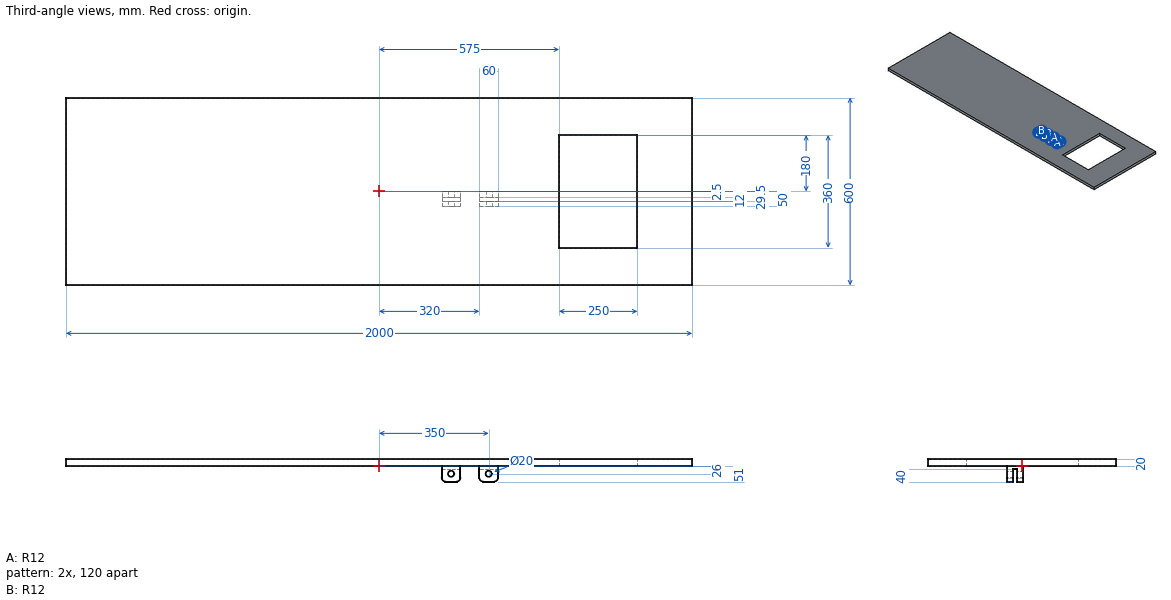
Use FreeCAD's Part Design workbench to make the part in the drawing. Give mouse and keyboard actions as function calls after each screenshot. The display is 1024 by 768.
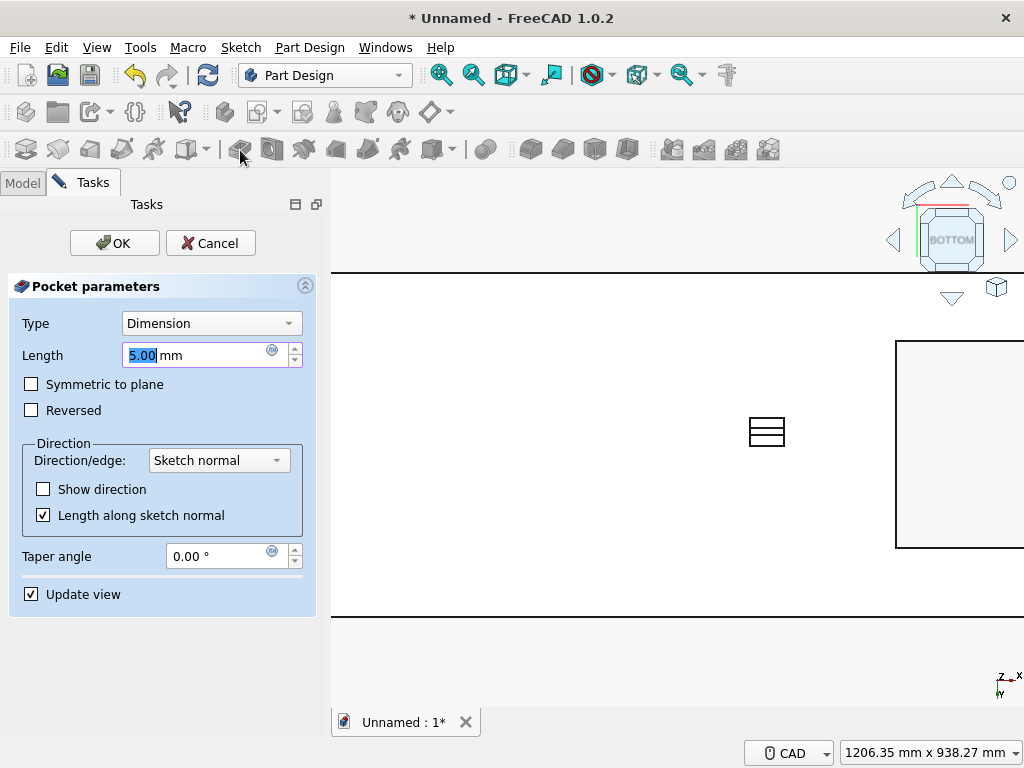
text(40)
key(Tab)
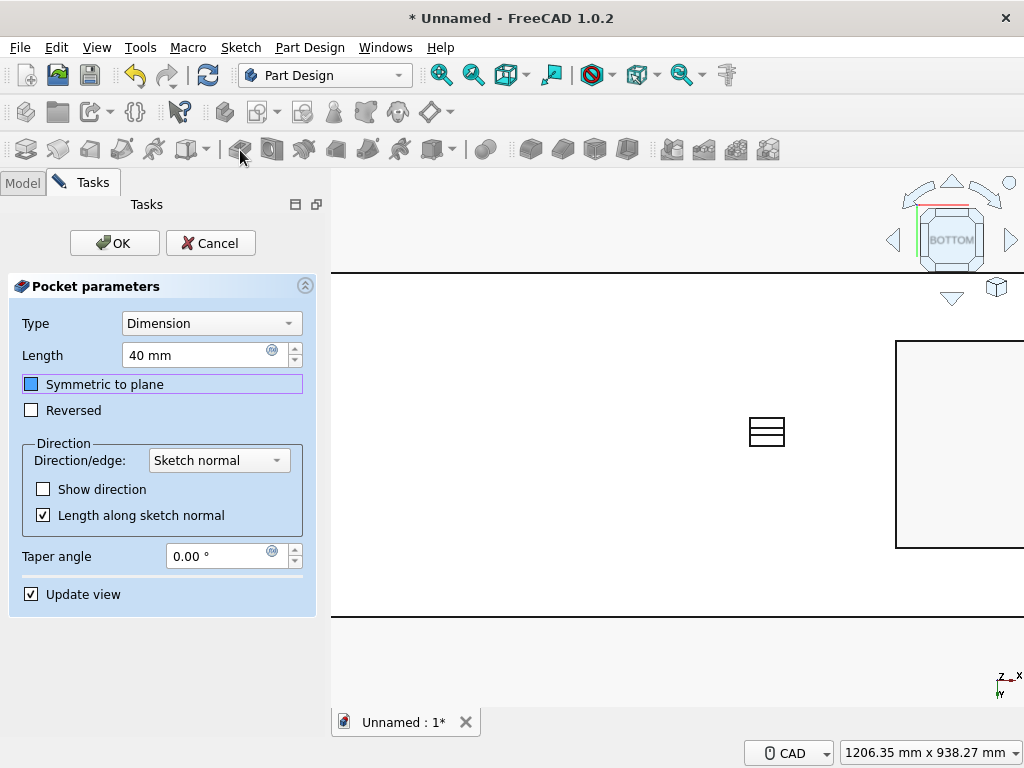
click(115, 243)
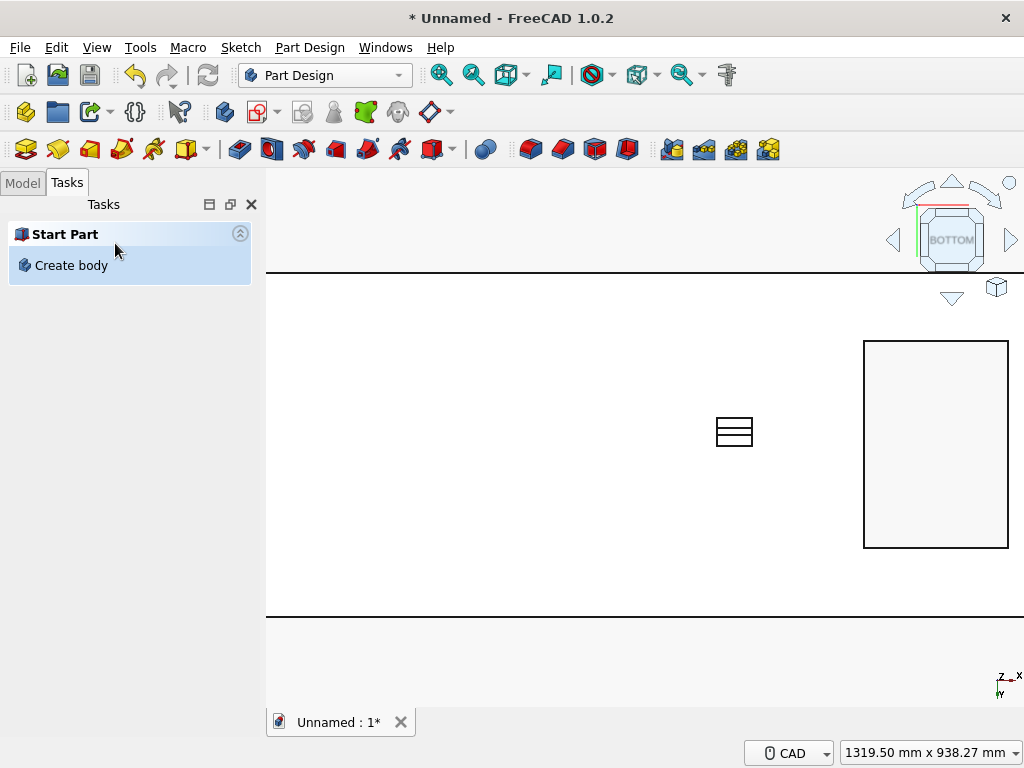
click(442, 76)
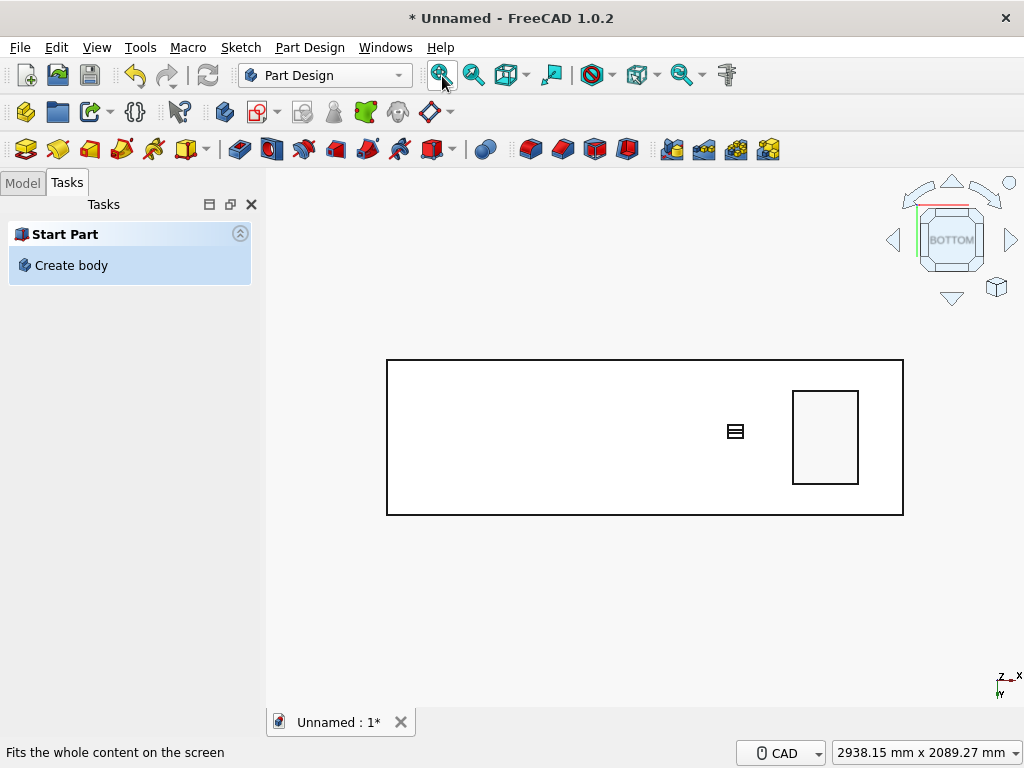
scroll(743, 435, up, 11)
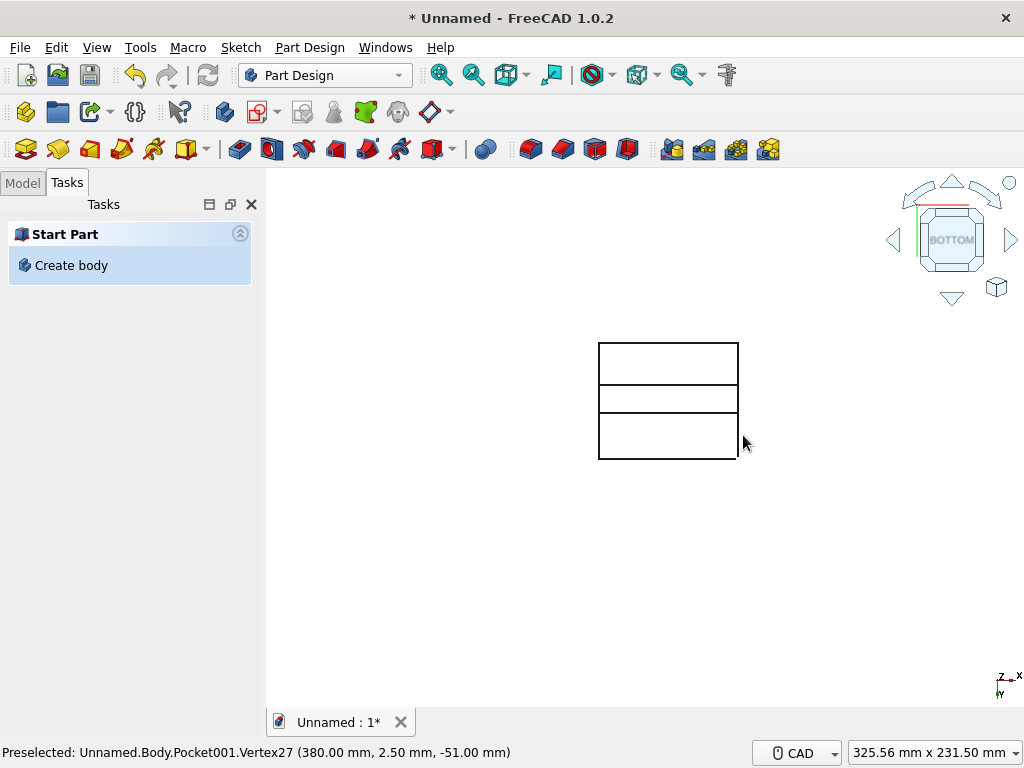
click(738, 435)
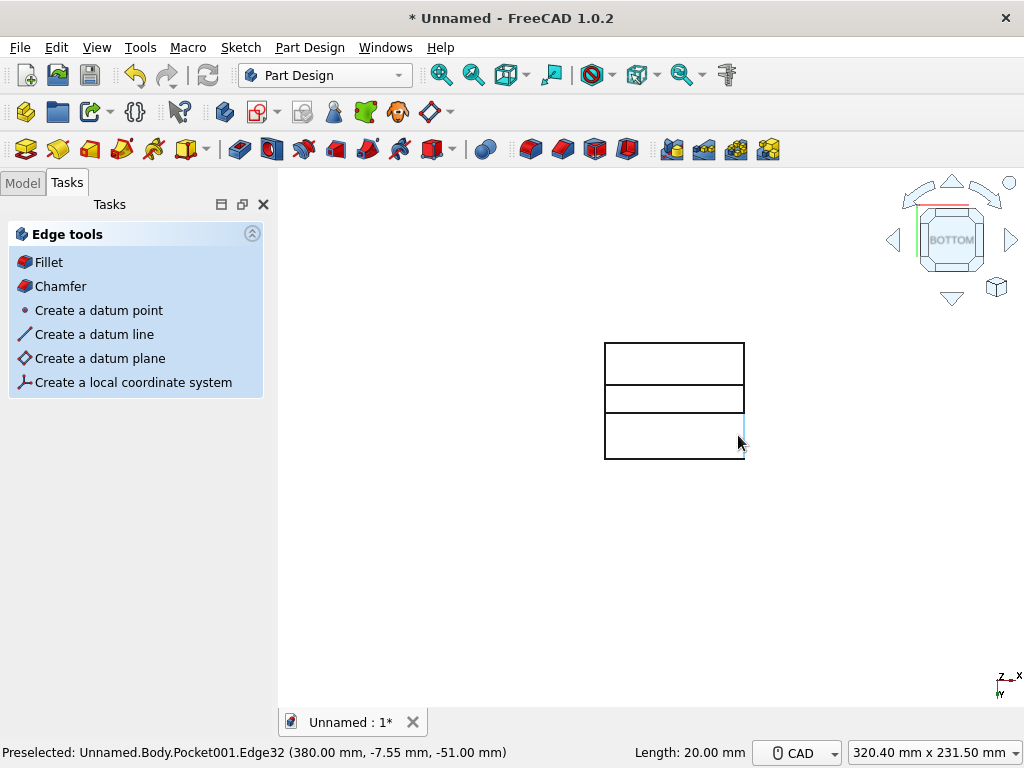
click(605, 363, ctrl)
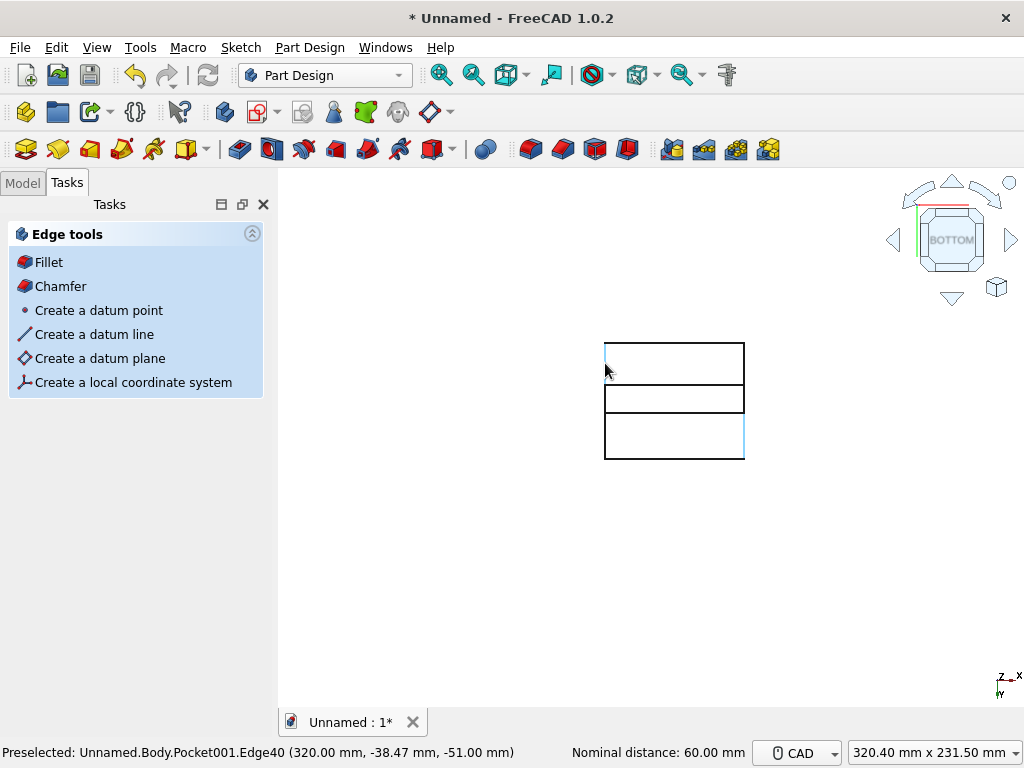
click(744, 363, ctrl)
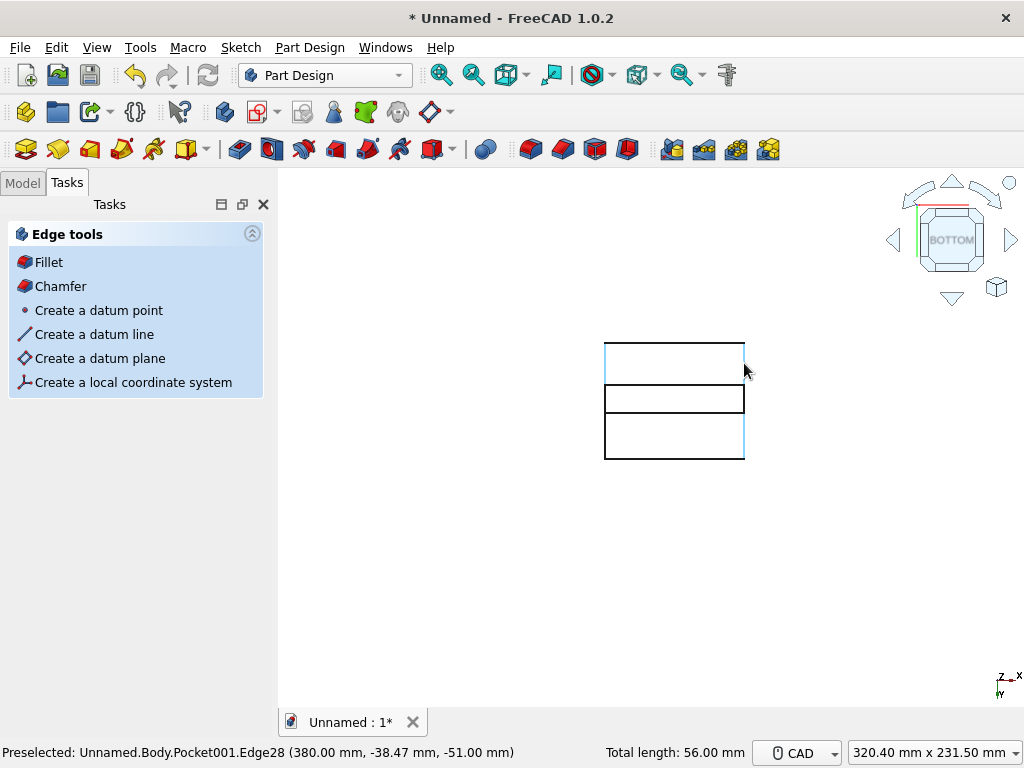
click(605, 435, ctrl)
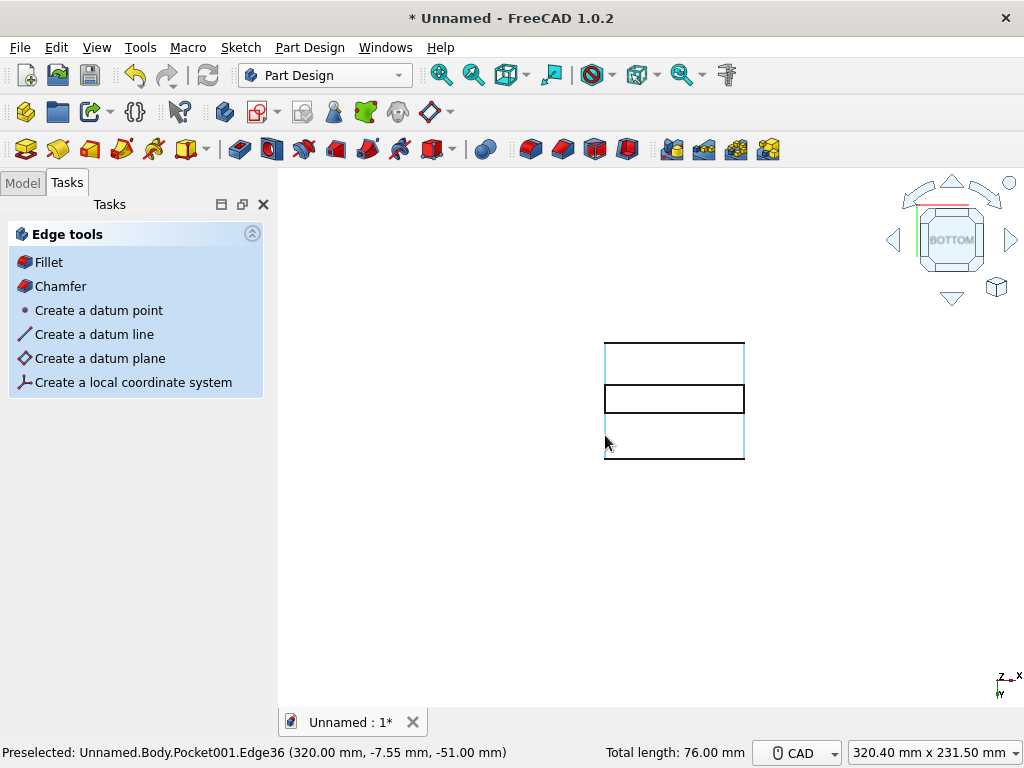
click(532, 150)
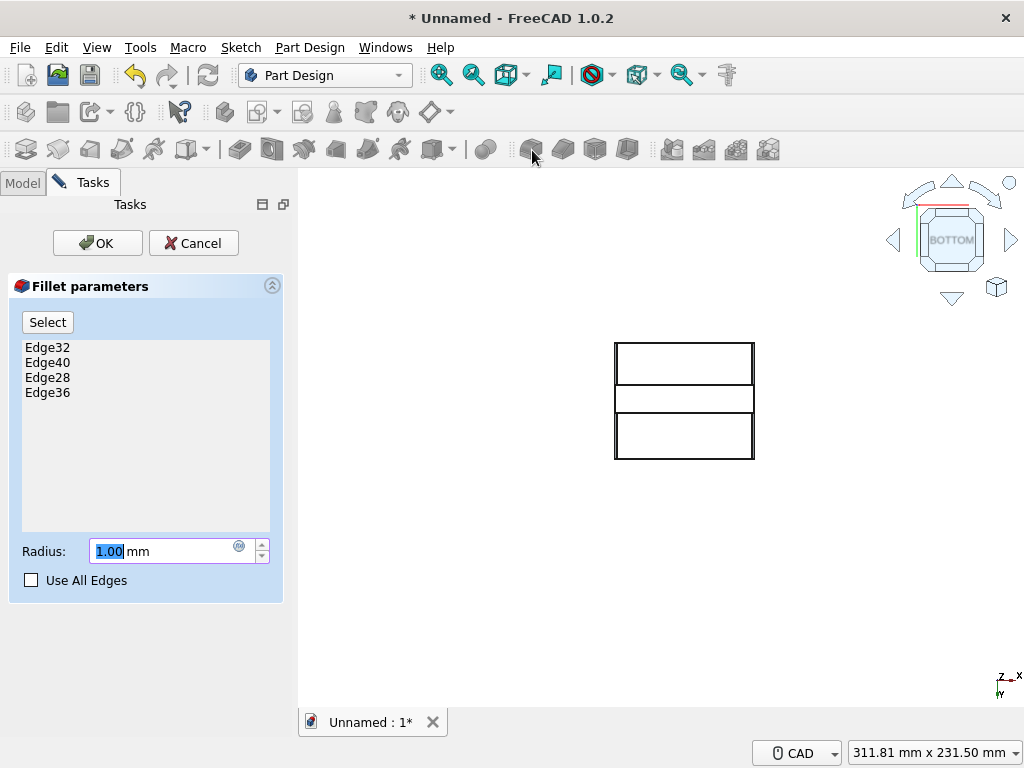
text(12)
key(Tab)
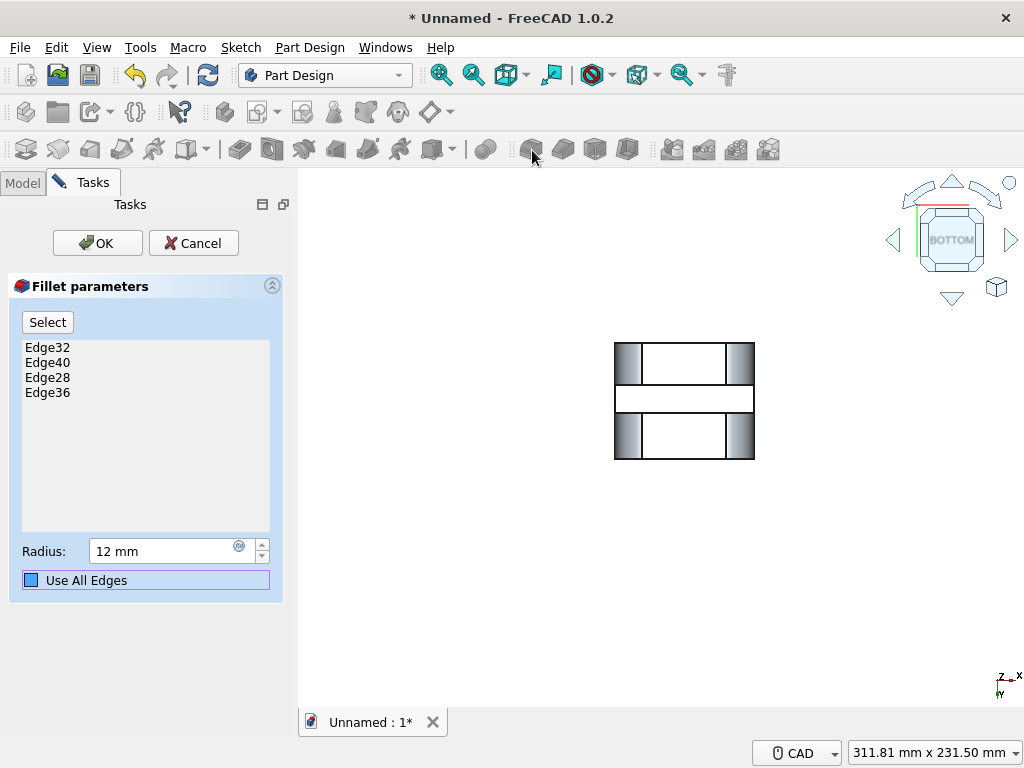
click(98, 243)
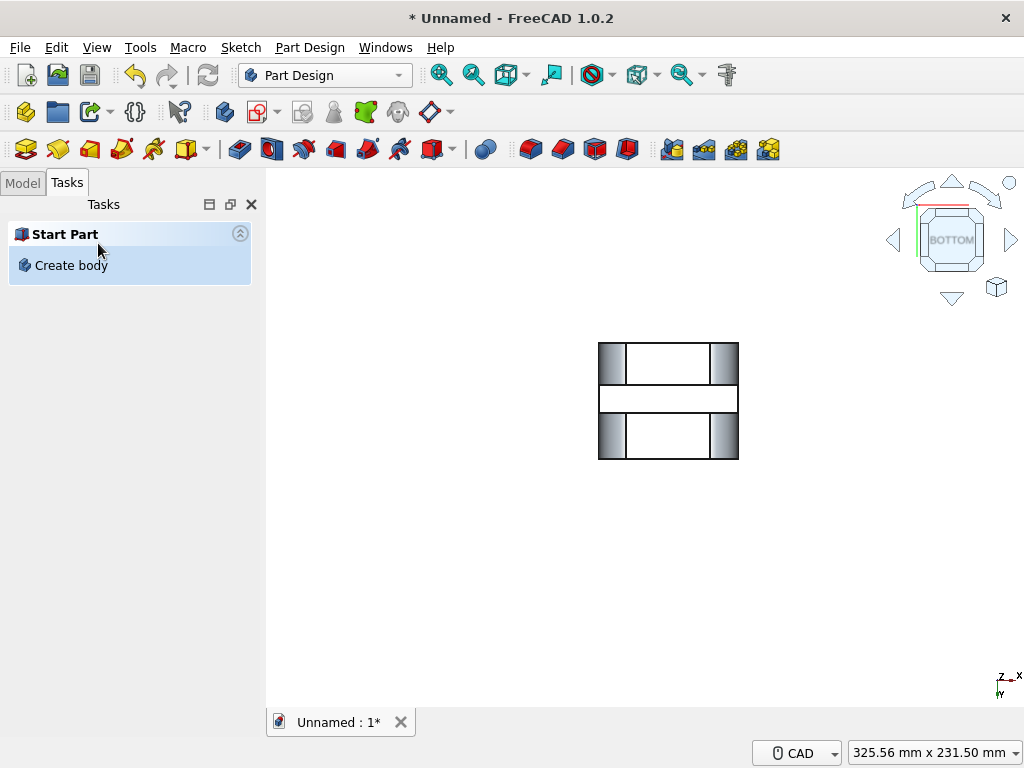
click(442, 76)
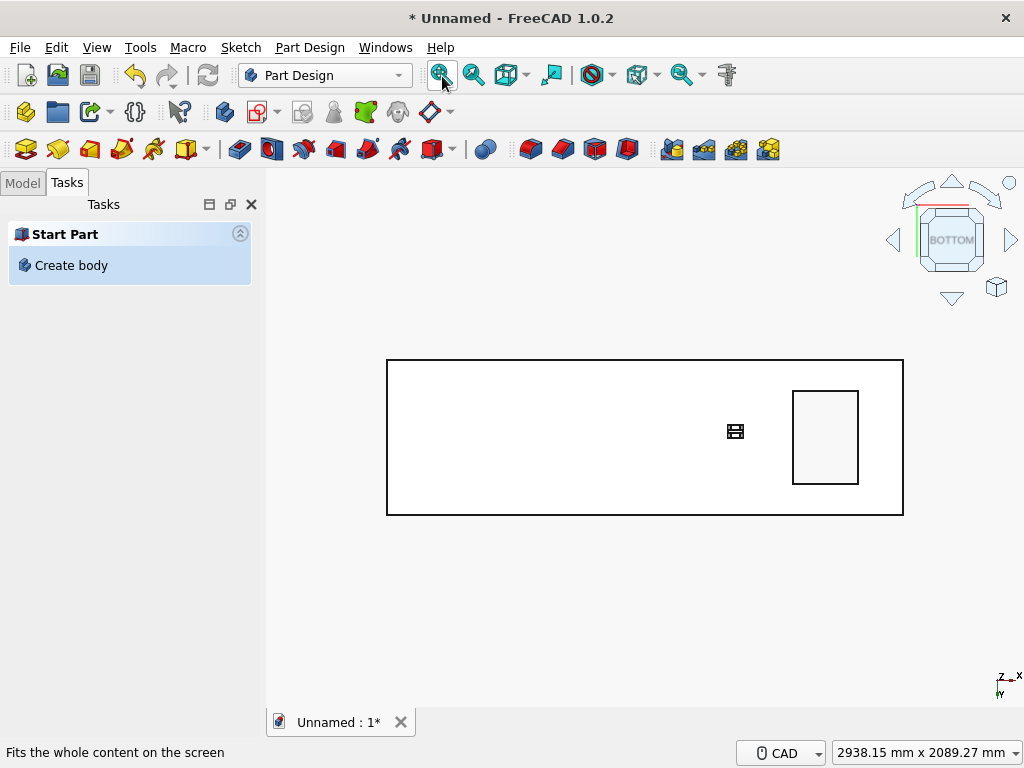
key(0)